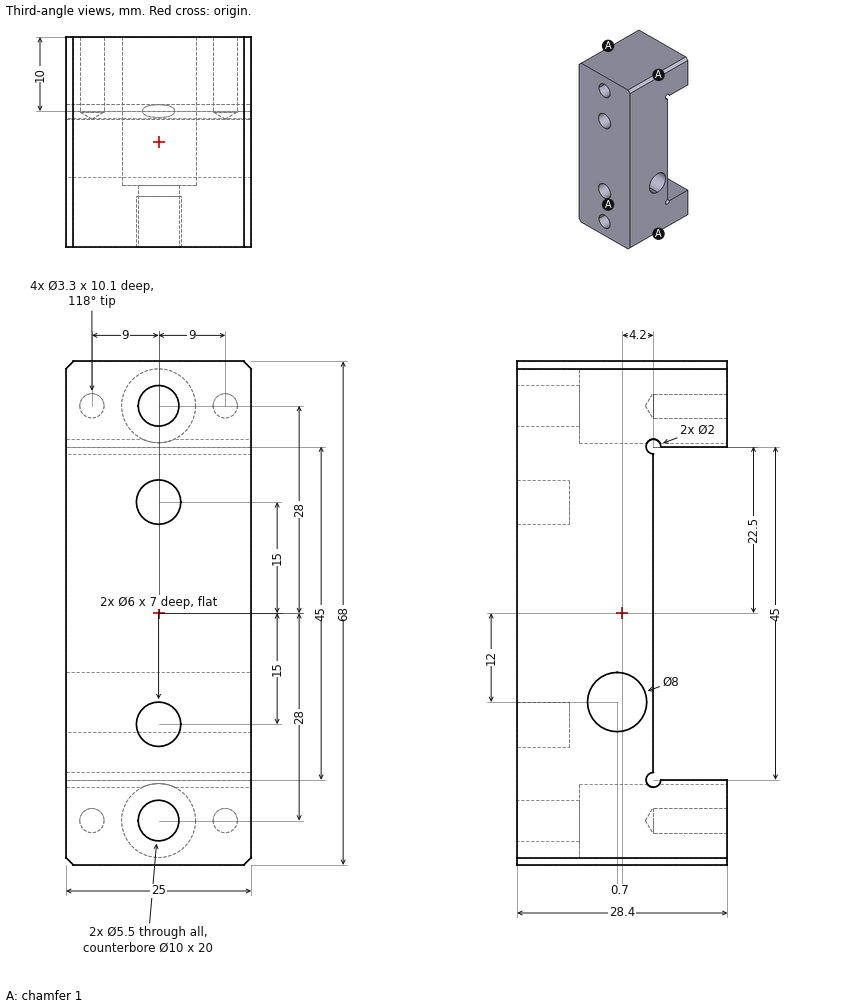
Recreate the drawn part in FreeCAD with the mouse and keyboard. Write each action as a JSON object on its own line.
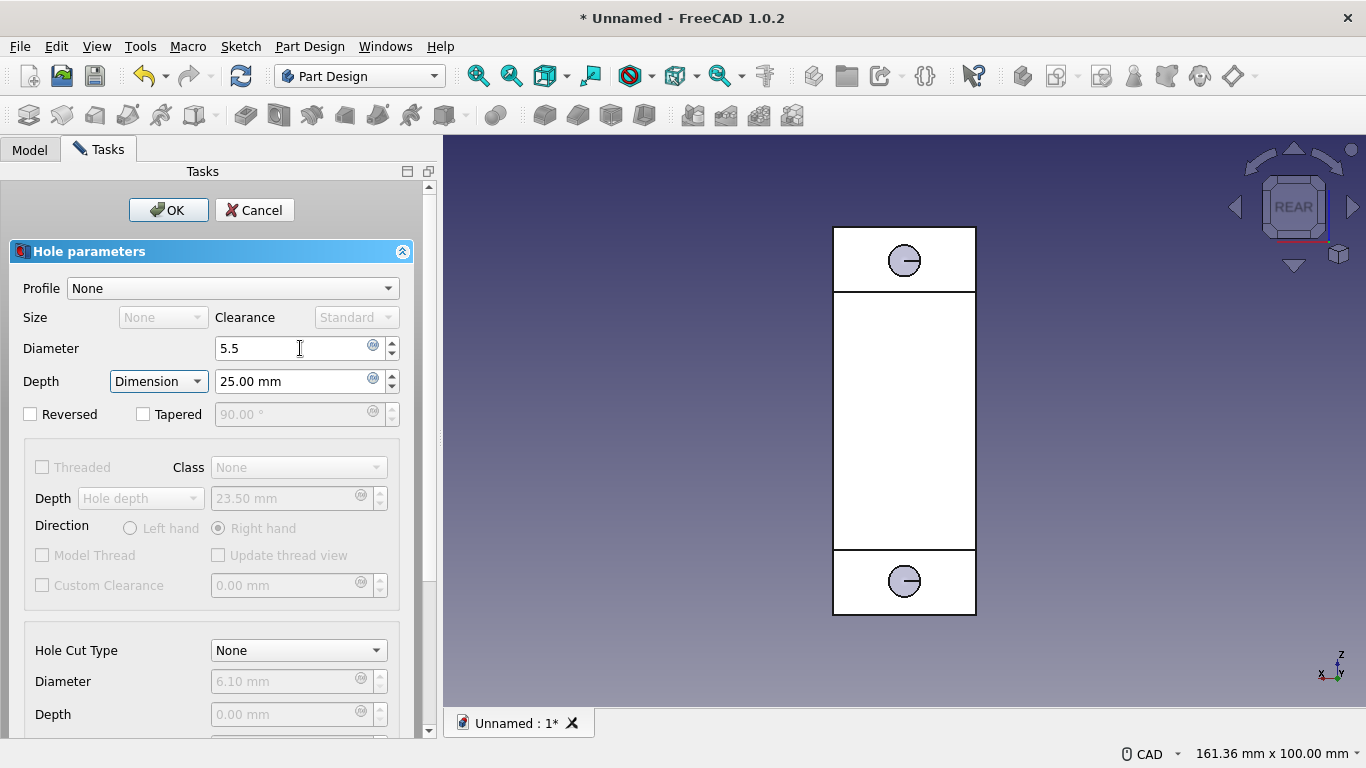
{"action": "left_click", "coordinate": [160, 382]}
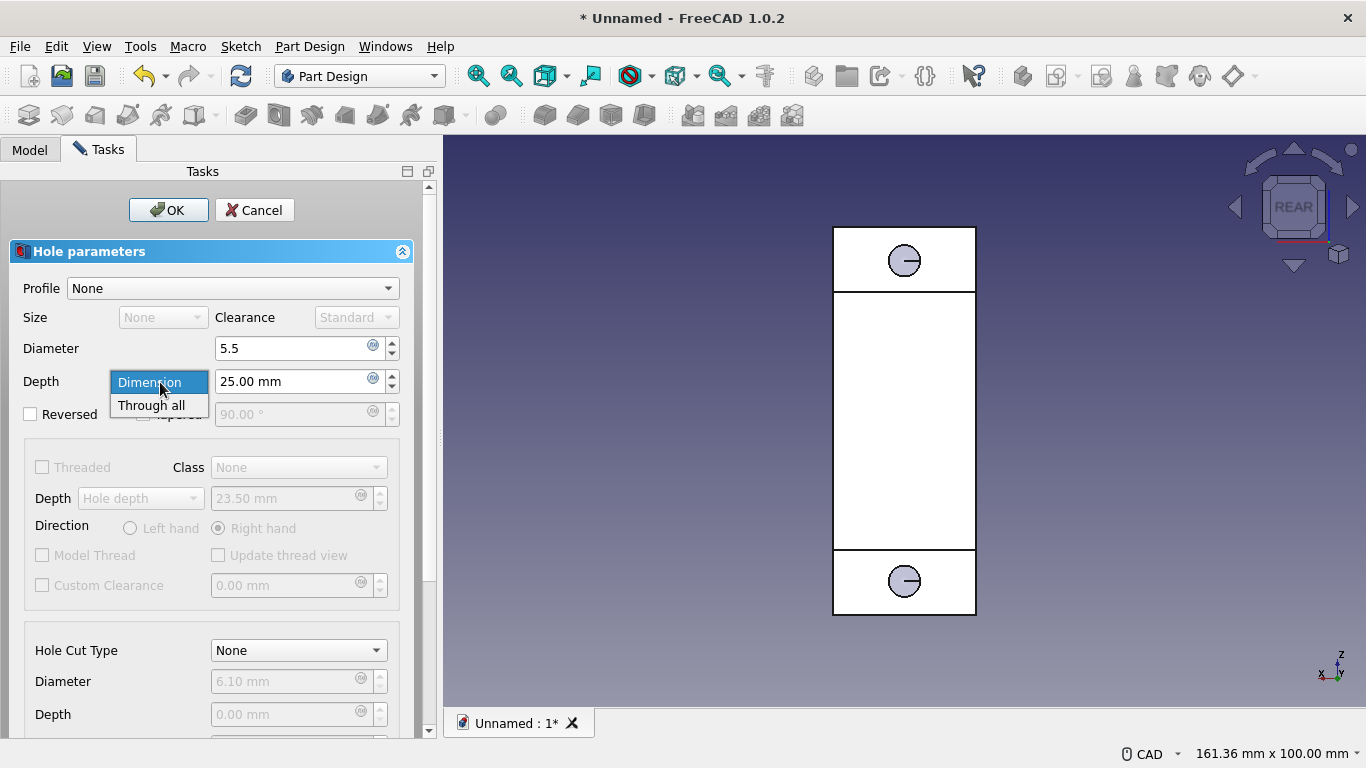
{"action": "left_click", "coordinate": [158, 406]}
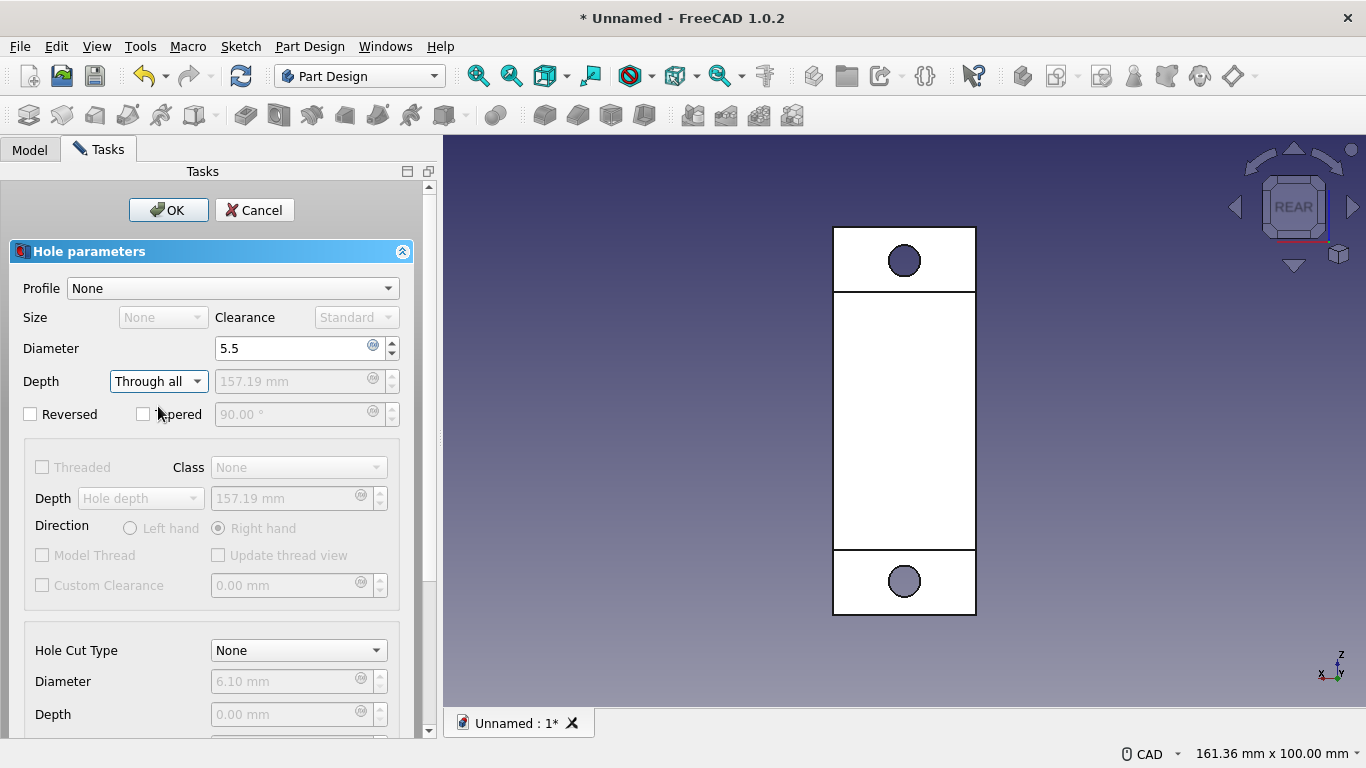
{"action": "left_click", "coordinate": [300, 650]}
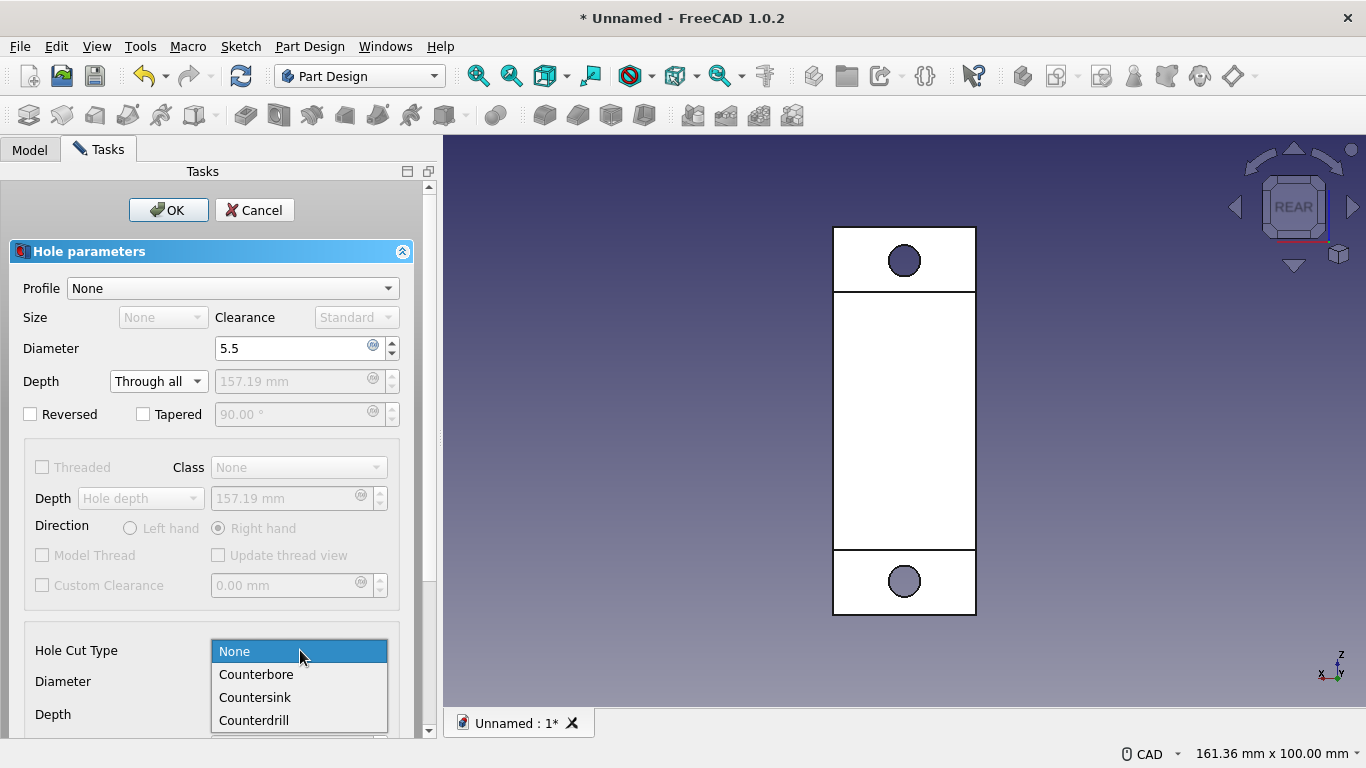
{"action": "left_click", "coordinate": [298, 674]}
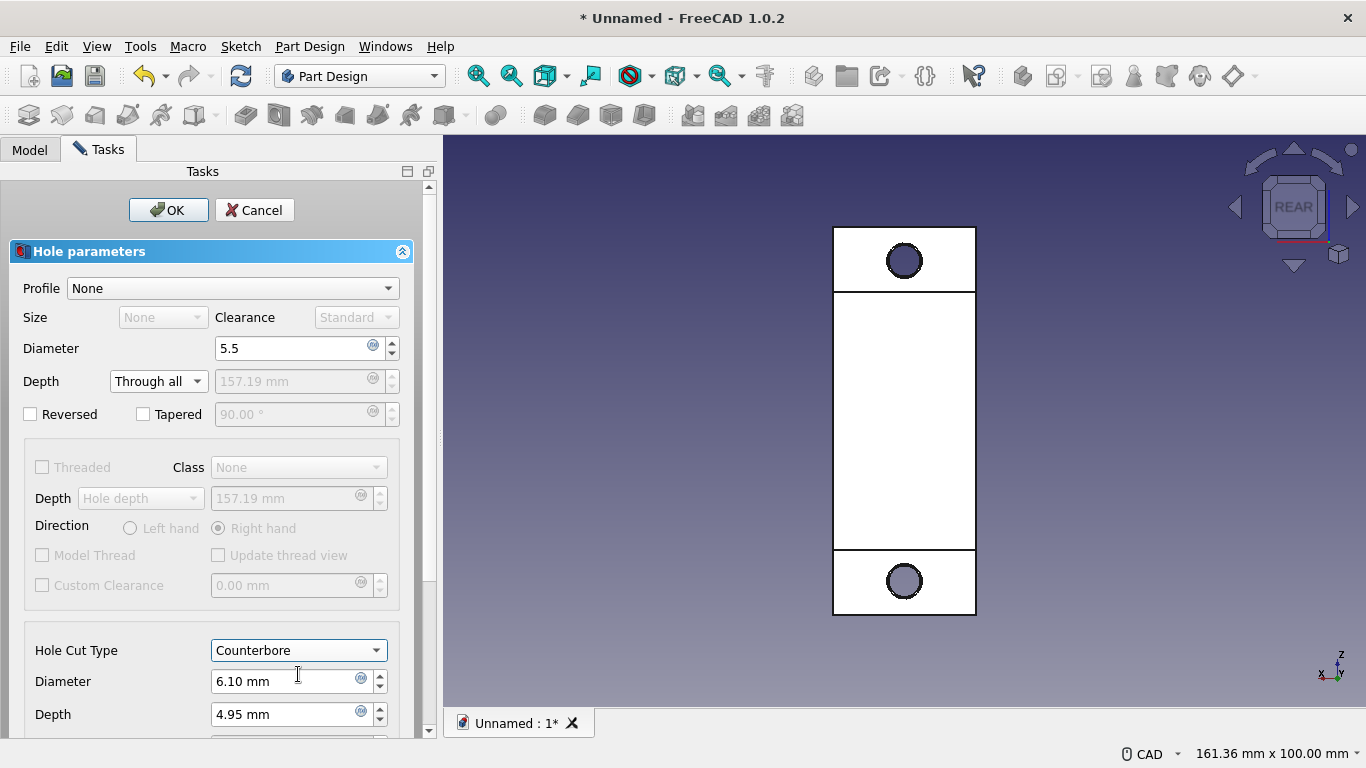
{"action": "triple_click", "coordinate": [292, 682]}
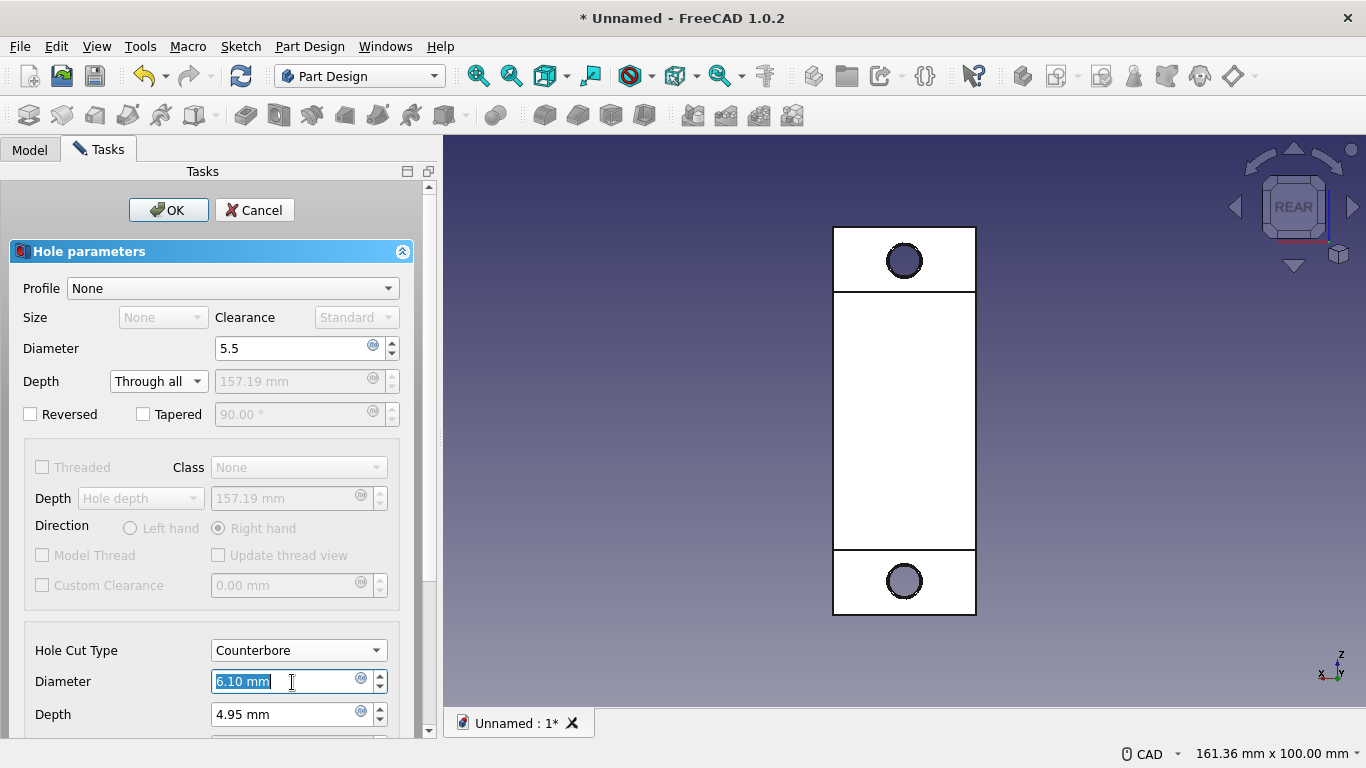
{"action": "type", "text": "10"}
{"action": "key", "text": "Tab"}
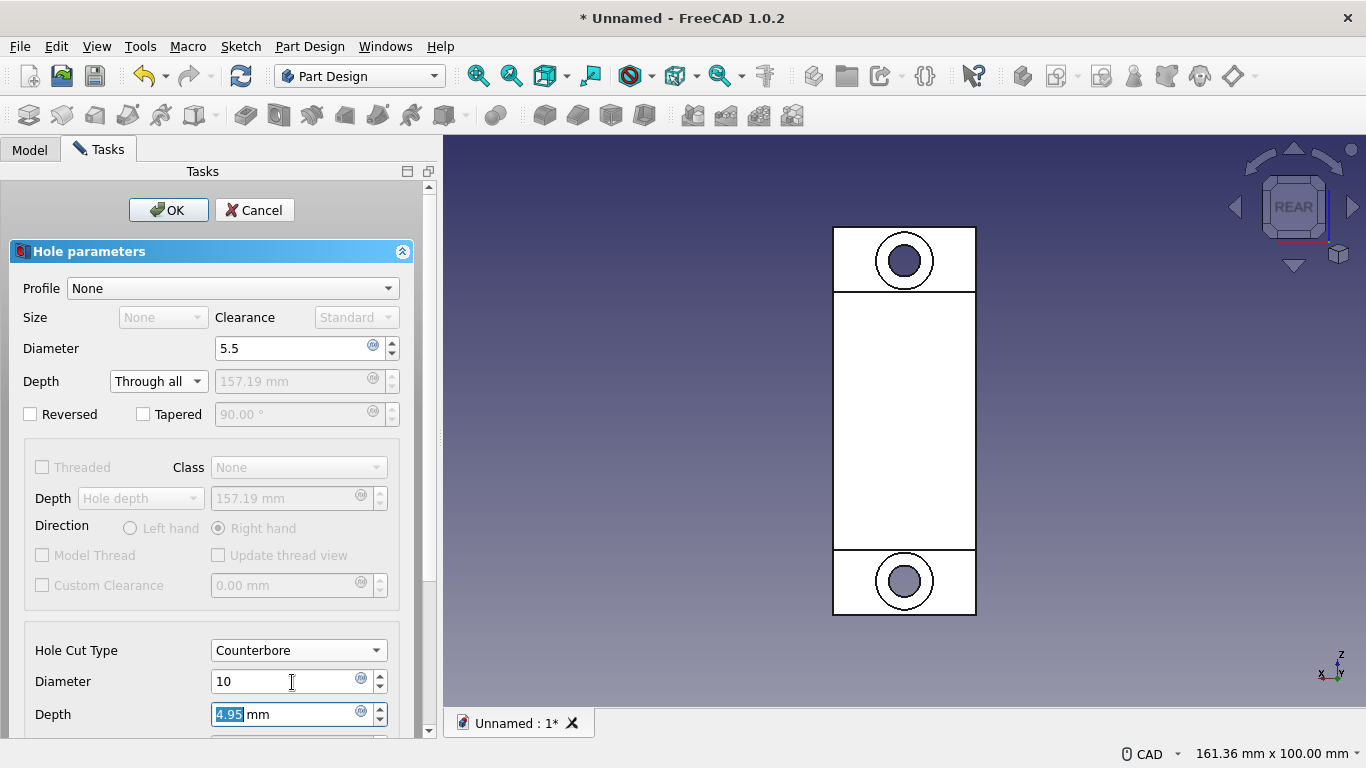
{"action": "type", "text": "20"}
{"action": "key", "text": "Tab"}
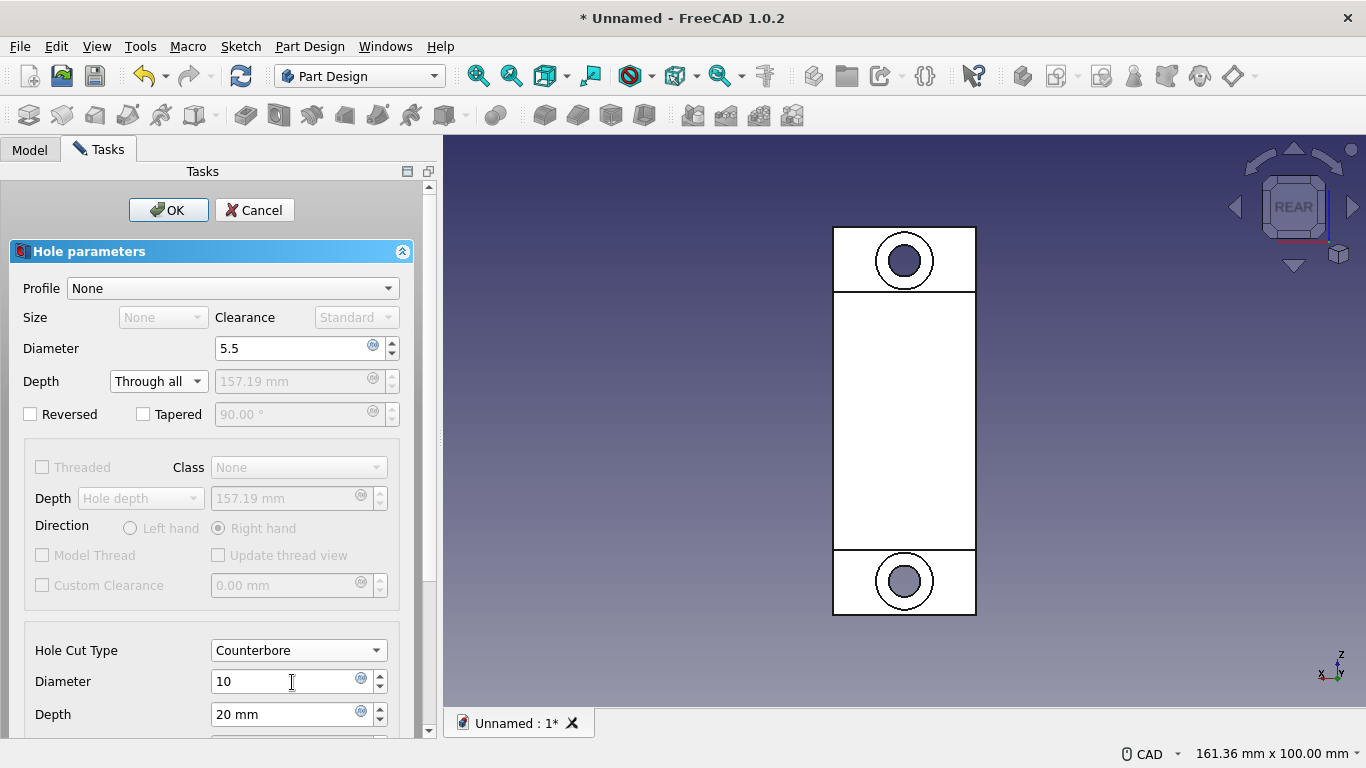
{"action": "left_click", "coordinate": [169, 210]}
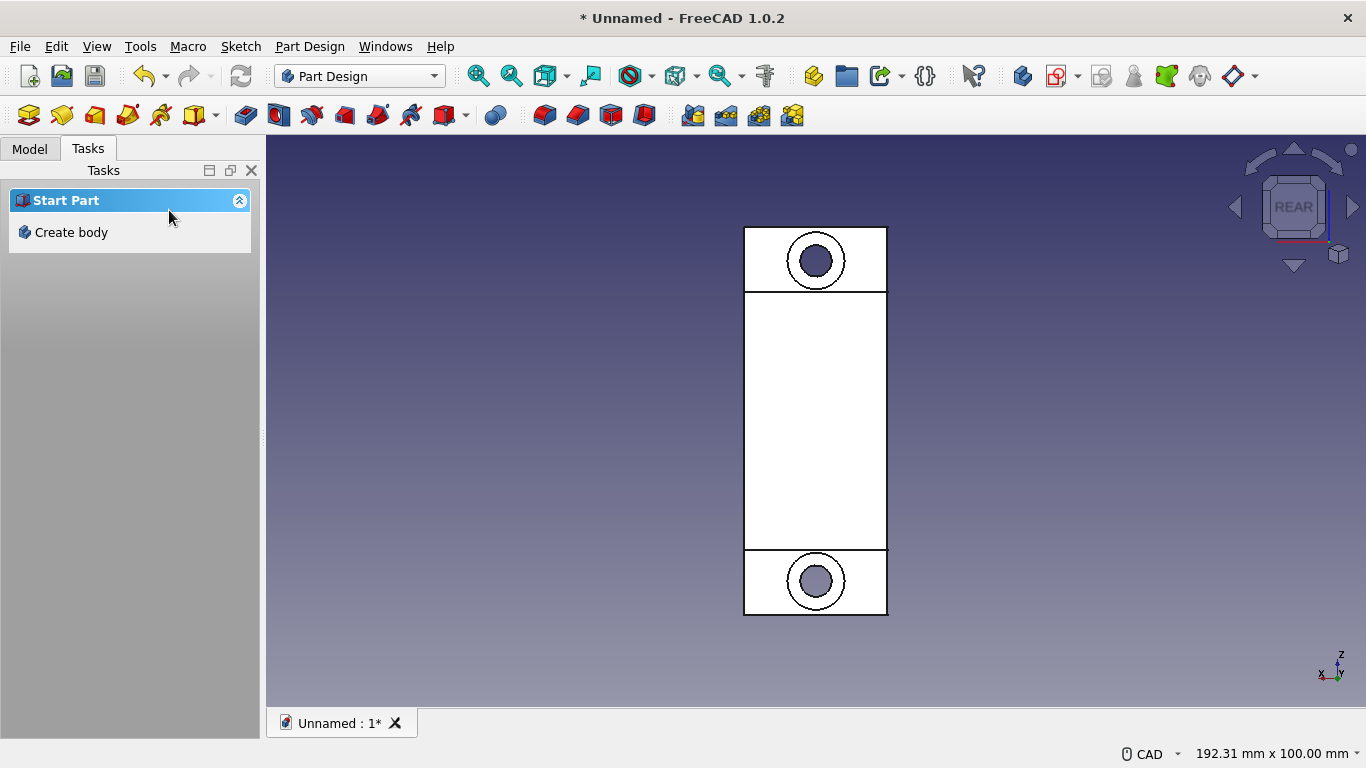
{"action": "left_click", "coordinate": [775, 563]}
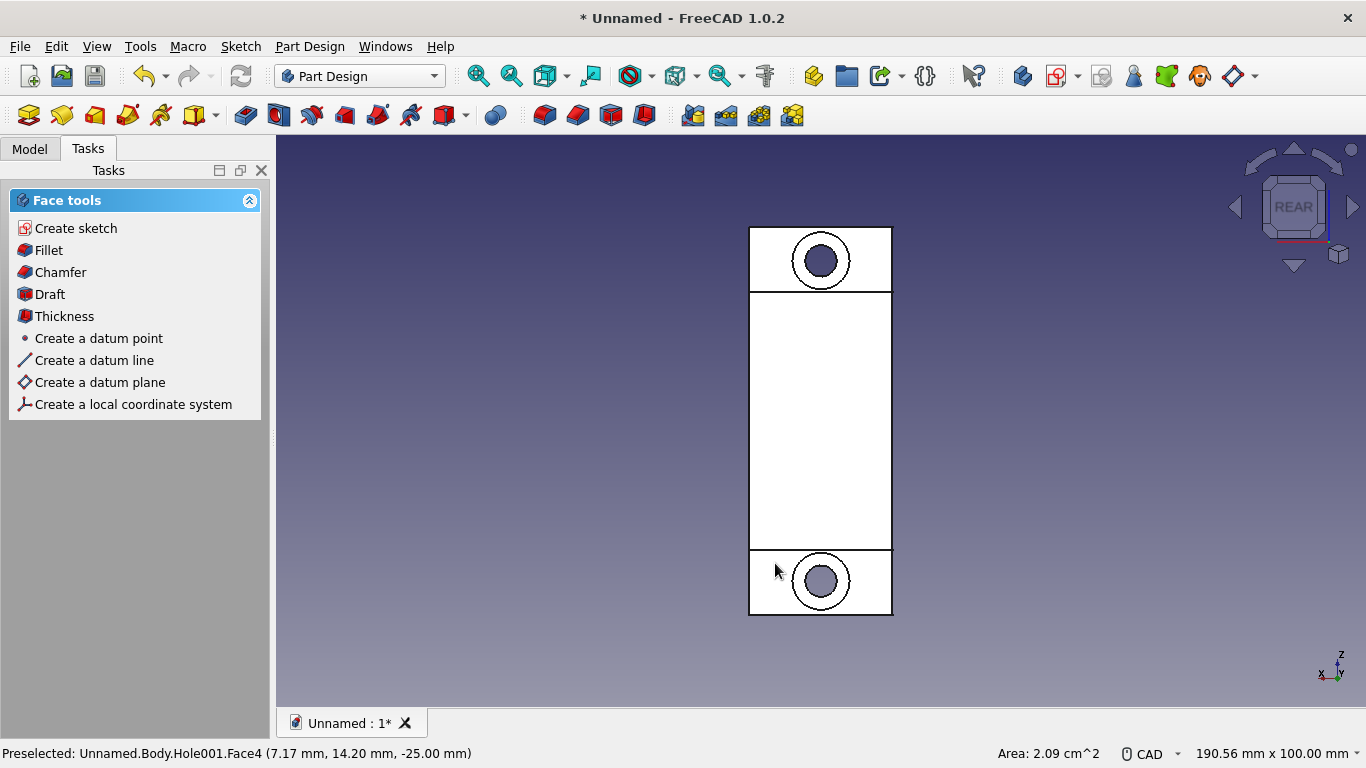
{"action": "left_click", "coordinate": [1056, 76]}